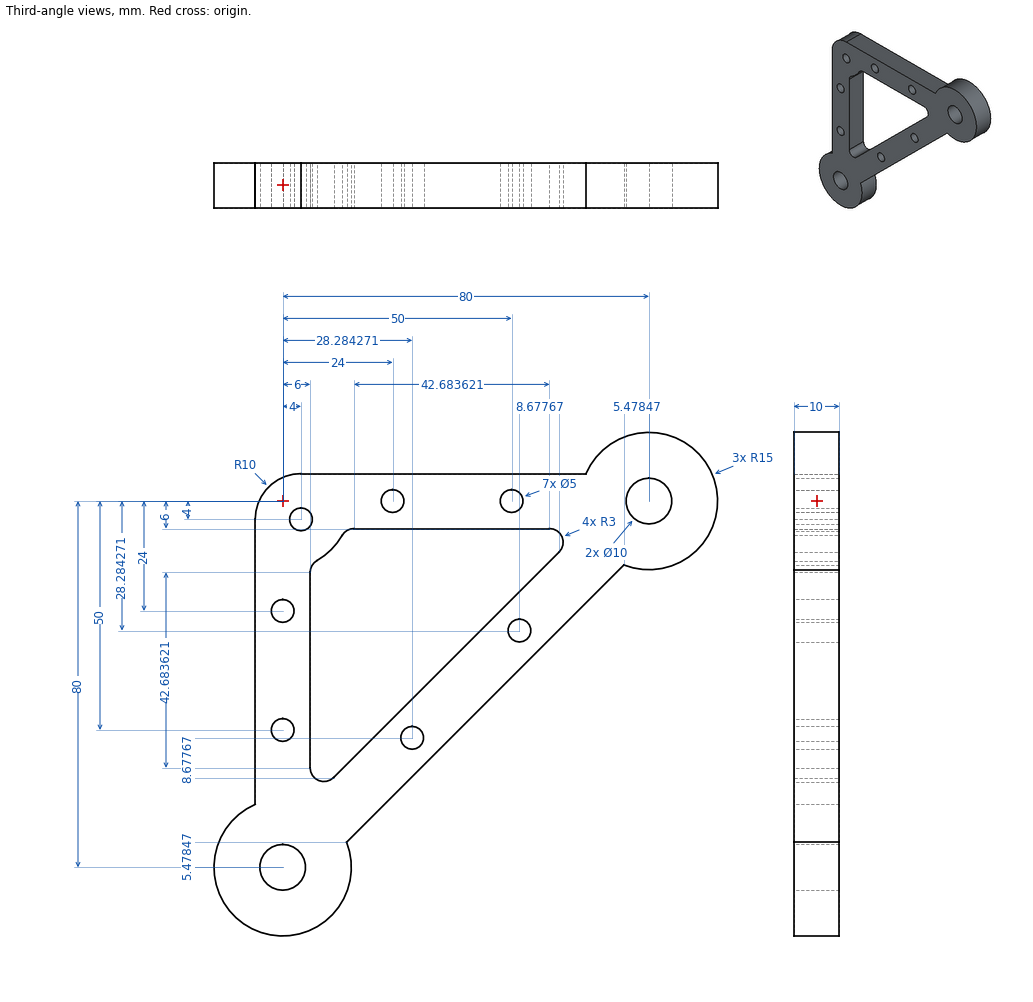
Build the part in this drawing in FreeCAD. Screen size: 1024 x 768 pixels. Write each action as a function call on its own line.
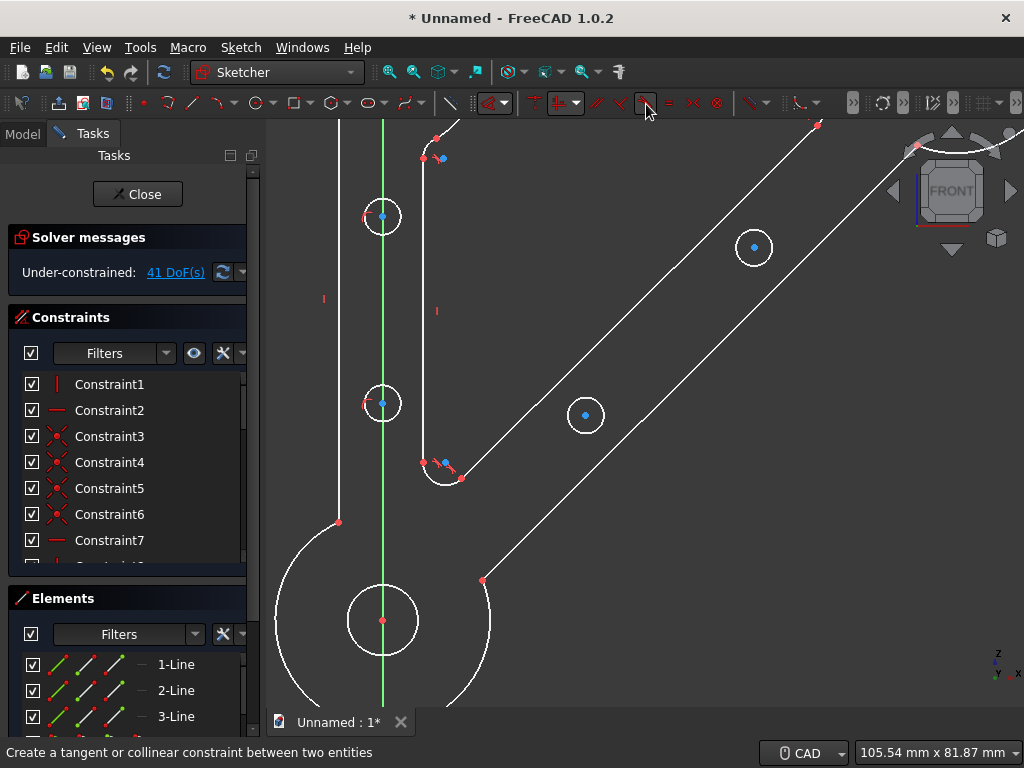
scroll(428, 478, down, 3)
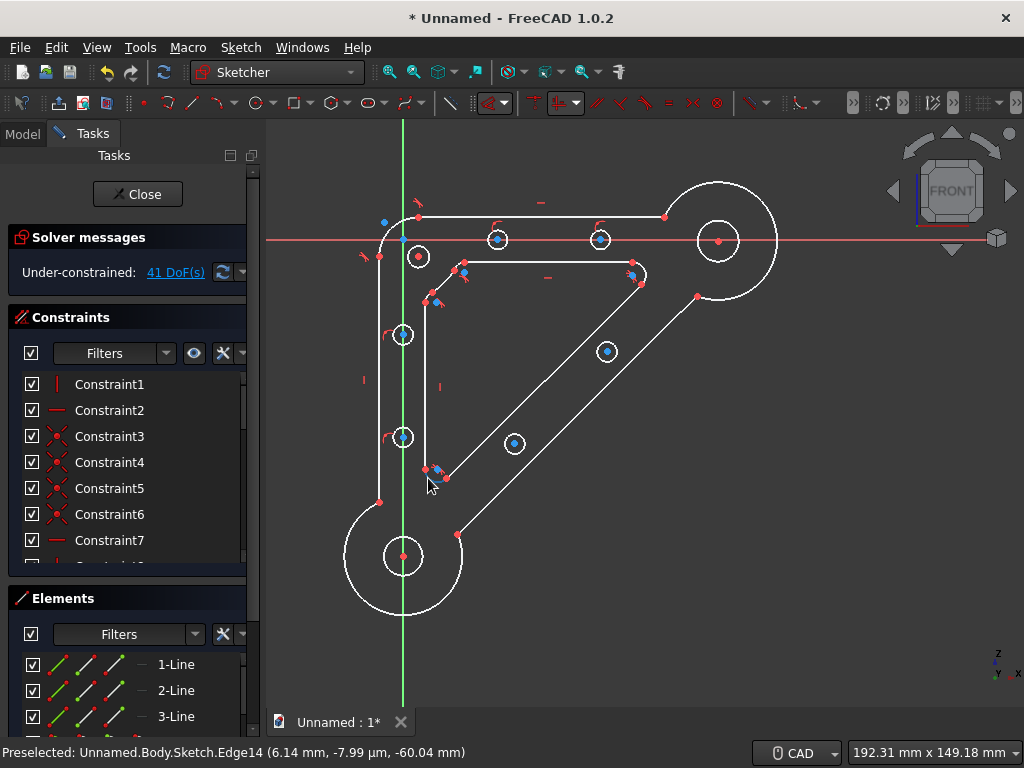
scroll(458, 265, up, 4)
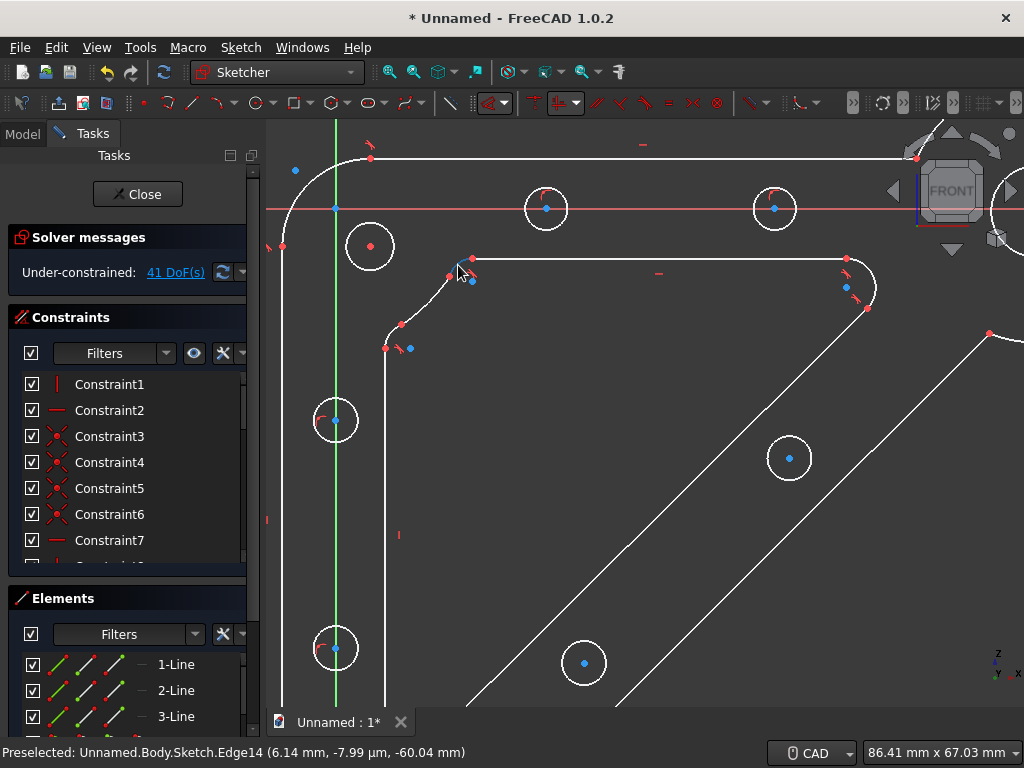
click(458, 264)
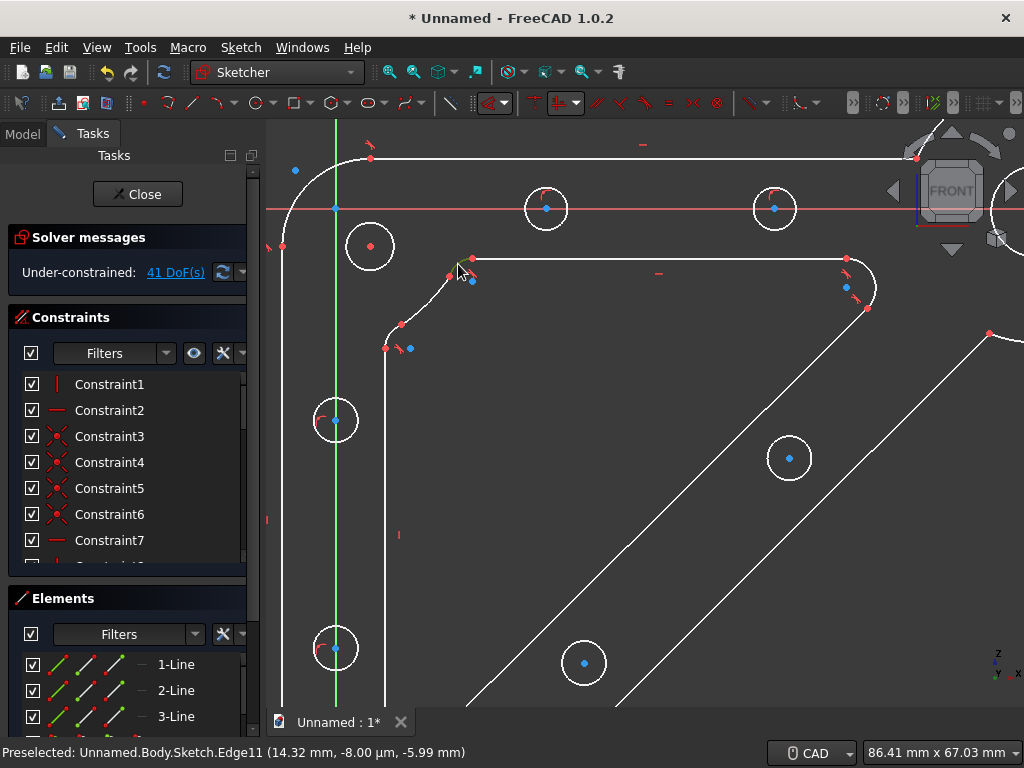
click(418, 312)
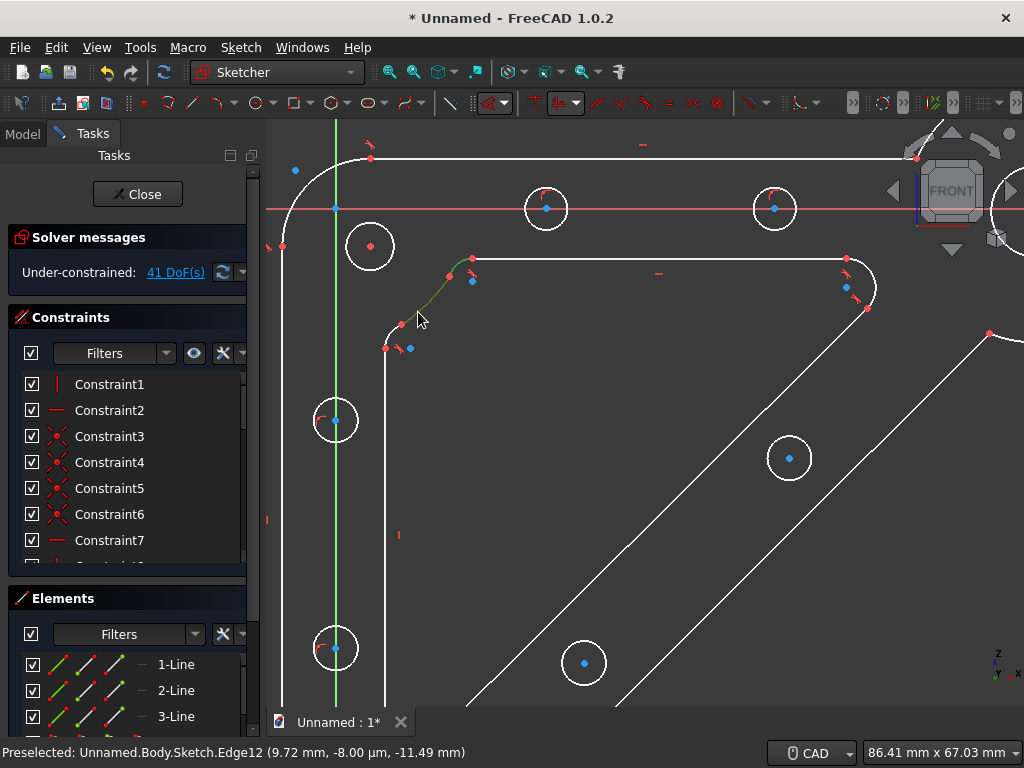
click(646, 104)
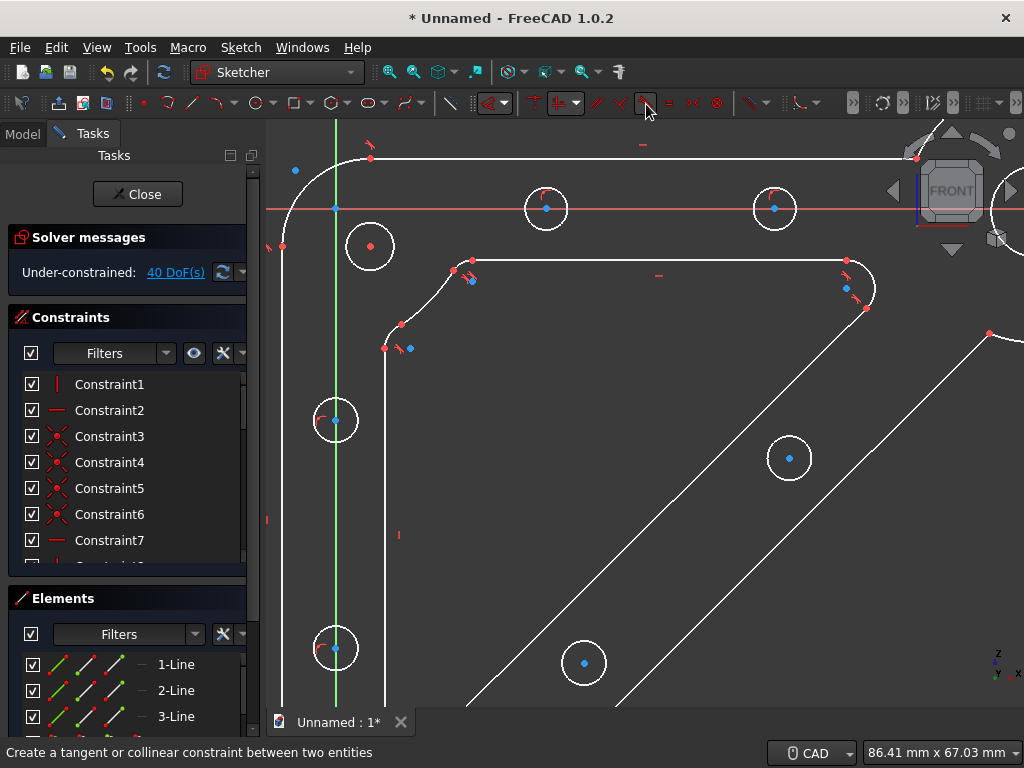
click(420, 311)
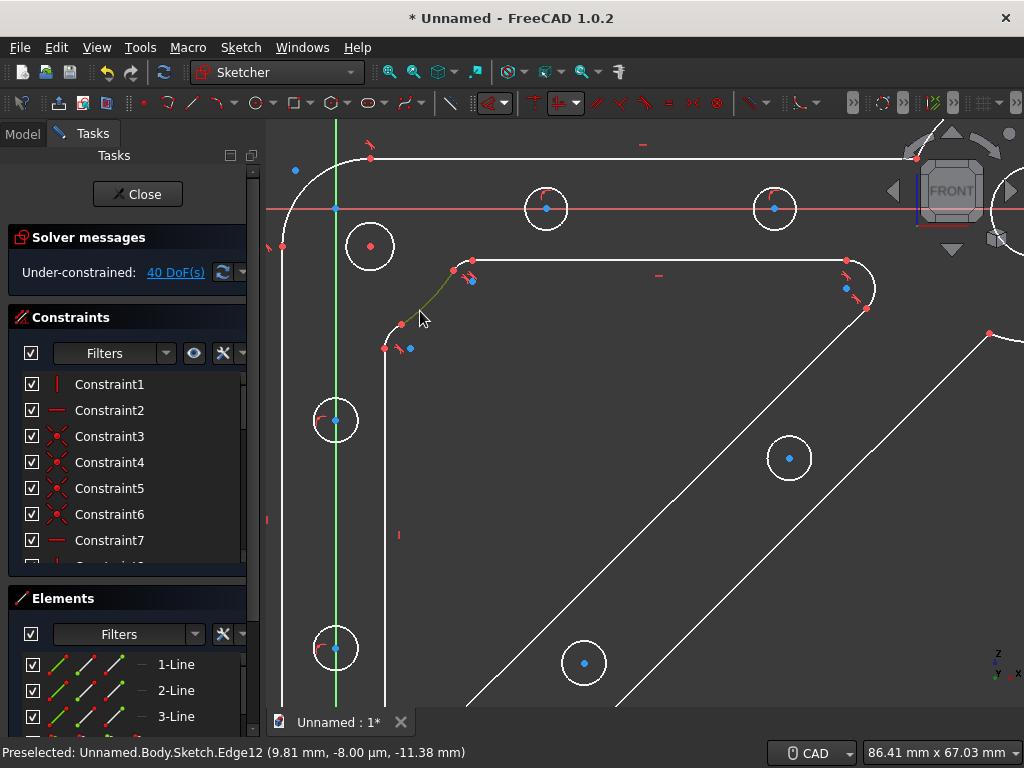
scroll(394, 329, up, 3)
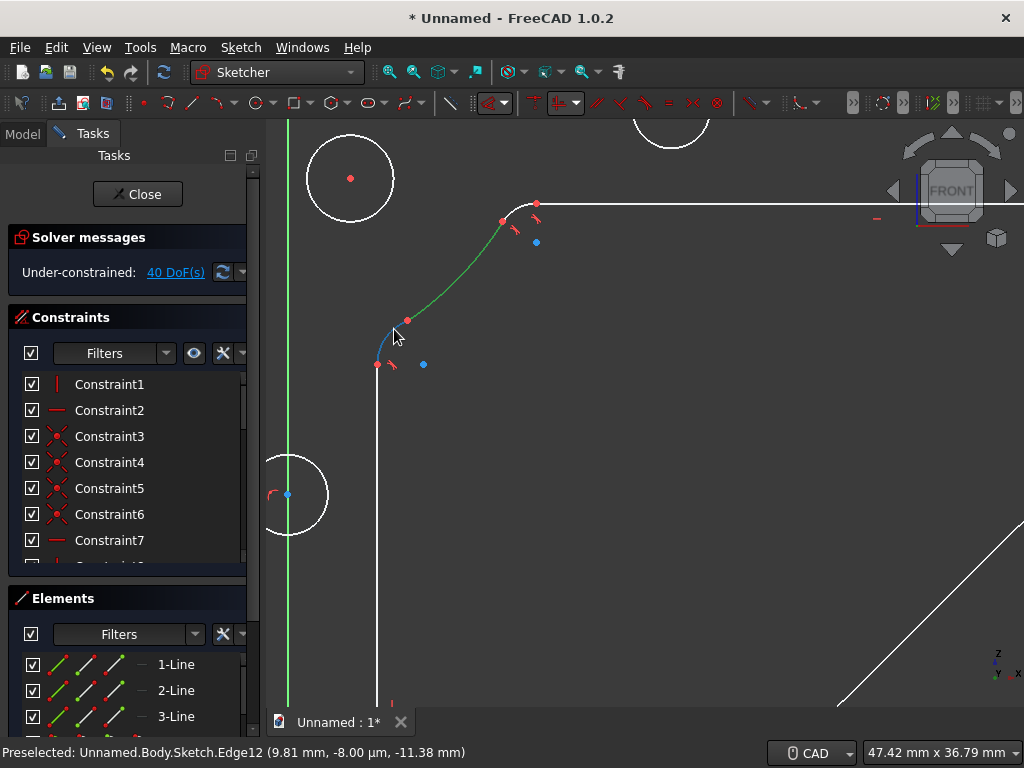
click(393, 329)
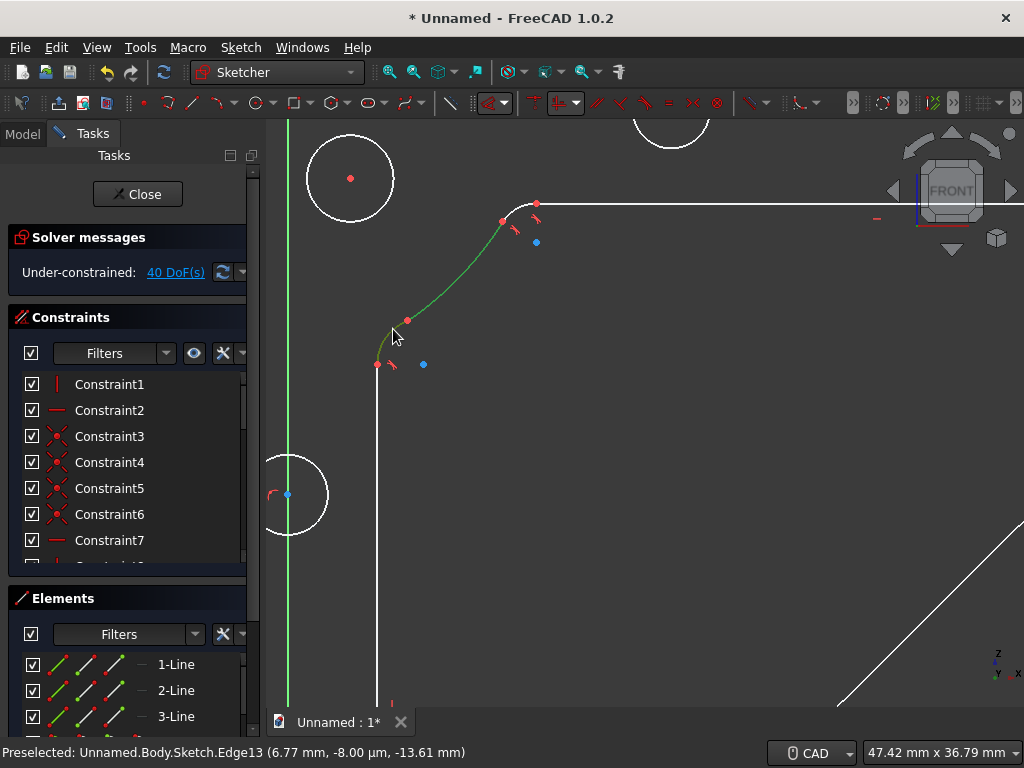
click(646, 104)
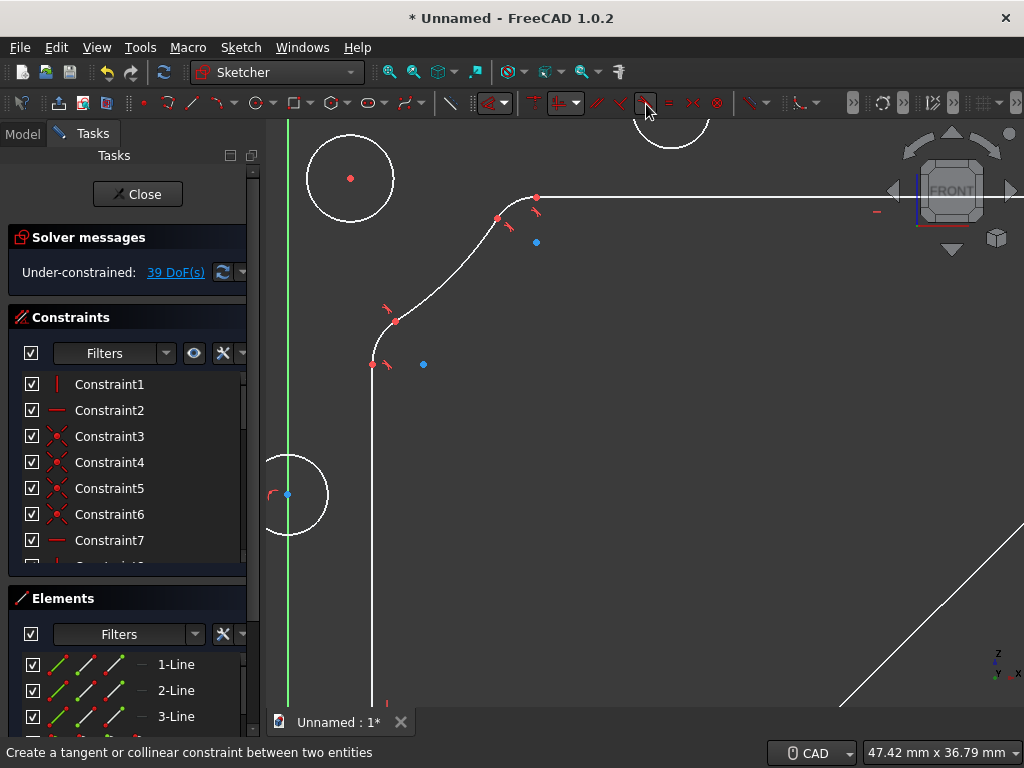
scroll(441, 282, down, 7)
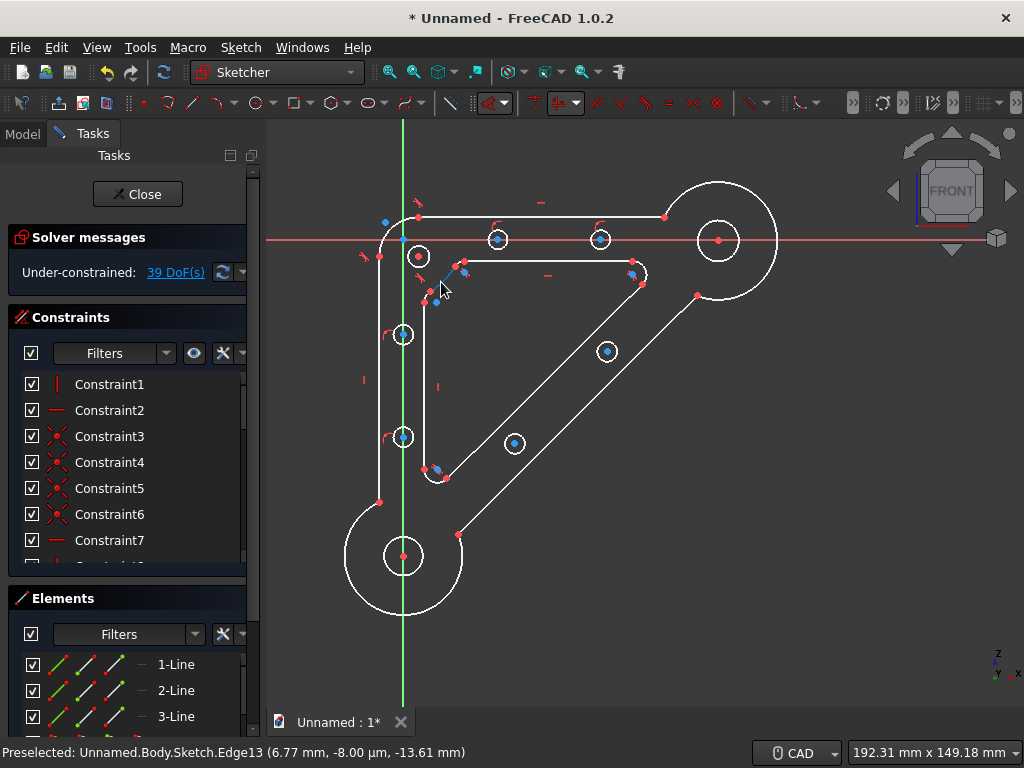
scroll(394, 231, up, 8)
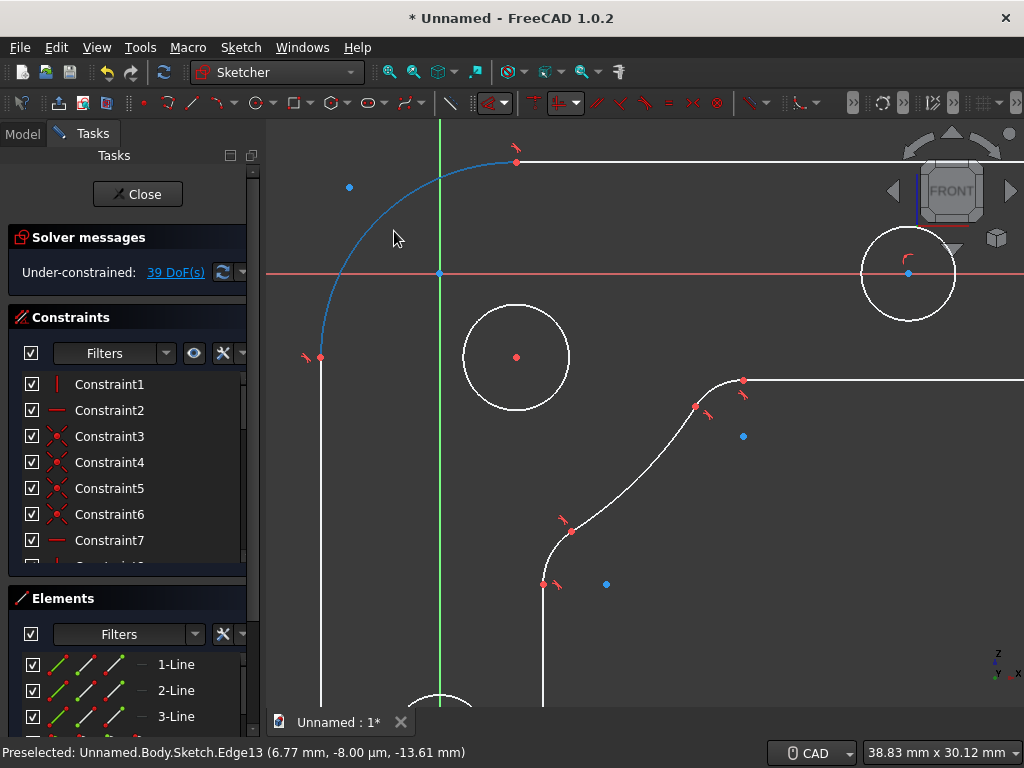
drag(339, 178, 450, 284)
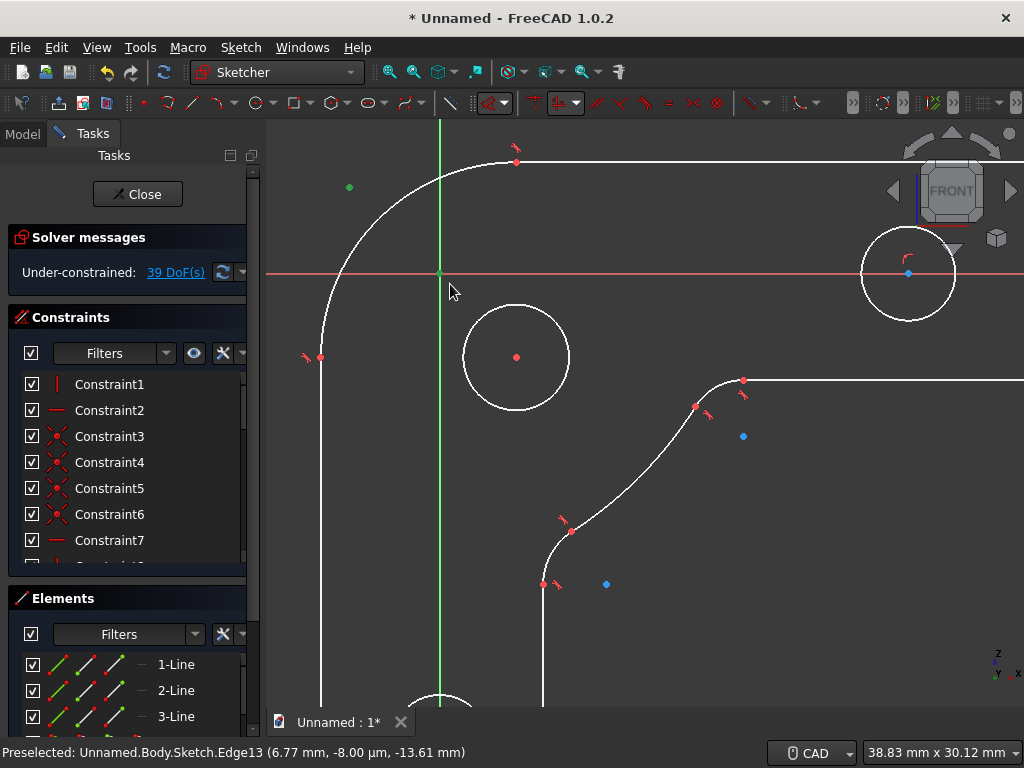
click(534, 104)